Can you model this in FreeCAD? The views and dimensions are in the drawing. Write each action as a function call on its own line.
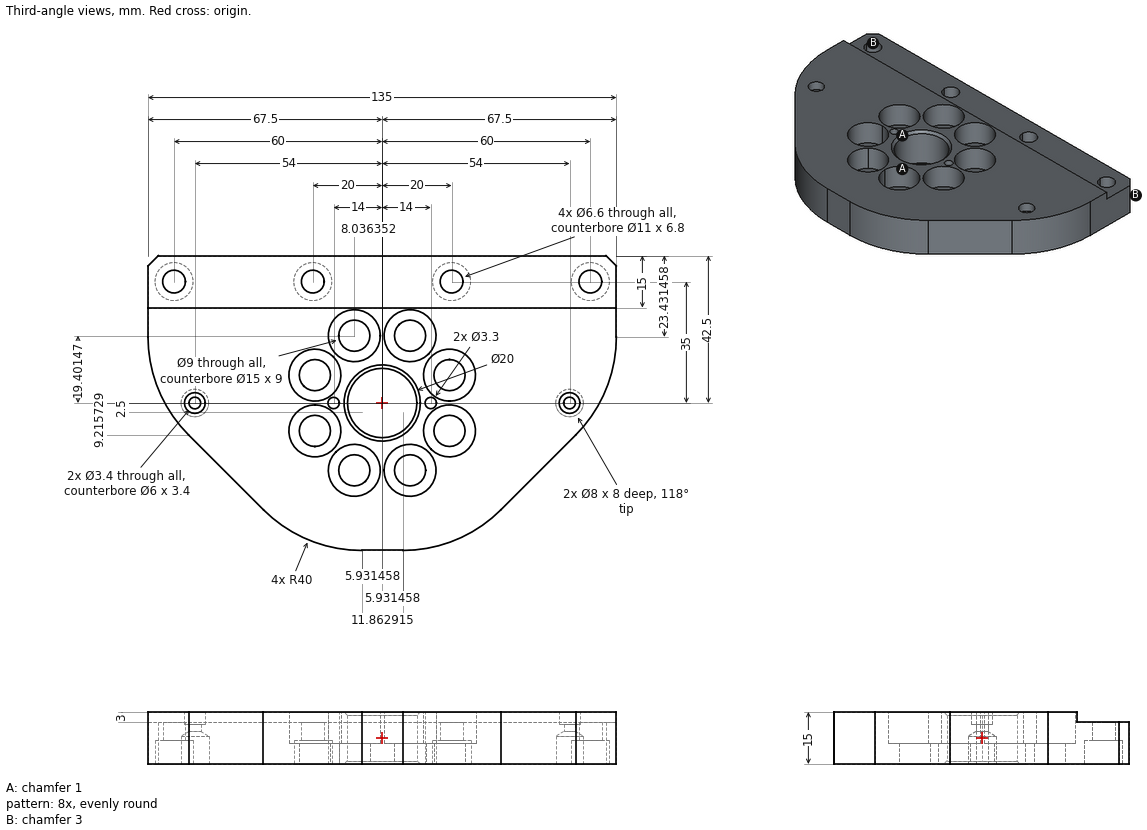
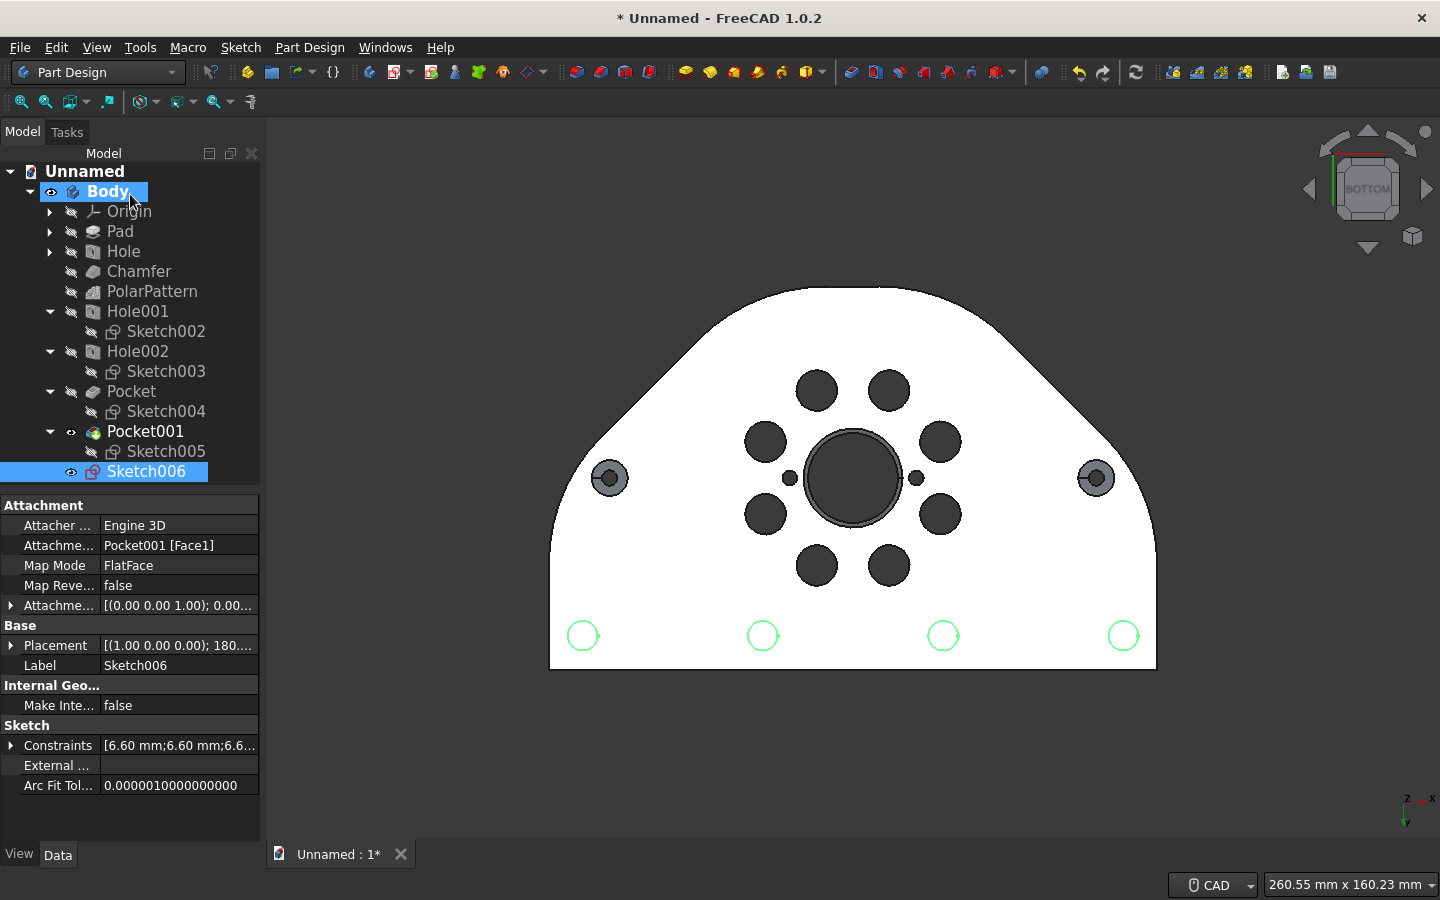
click(876, 72)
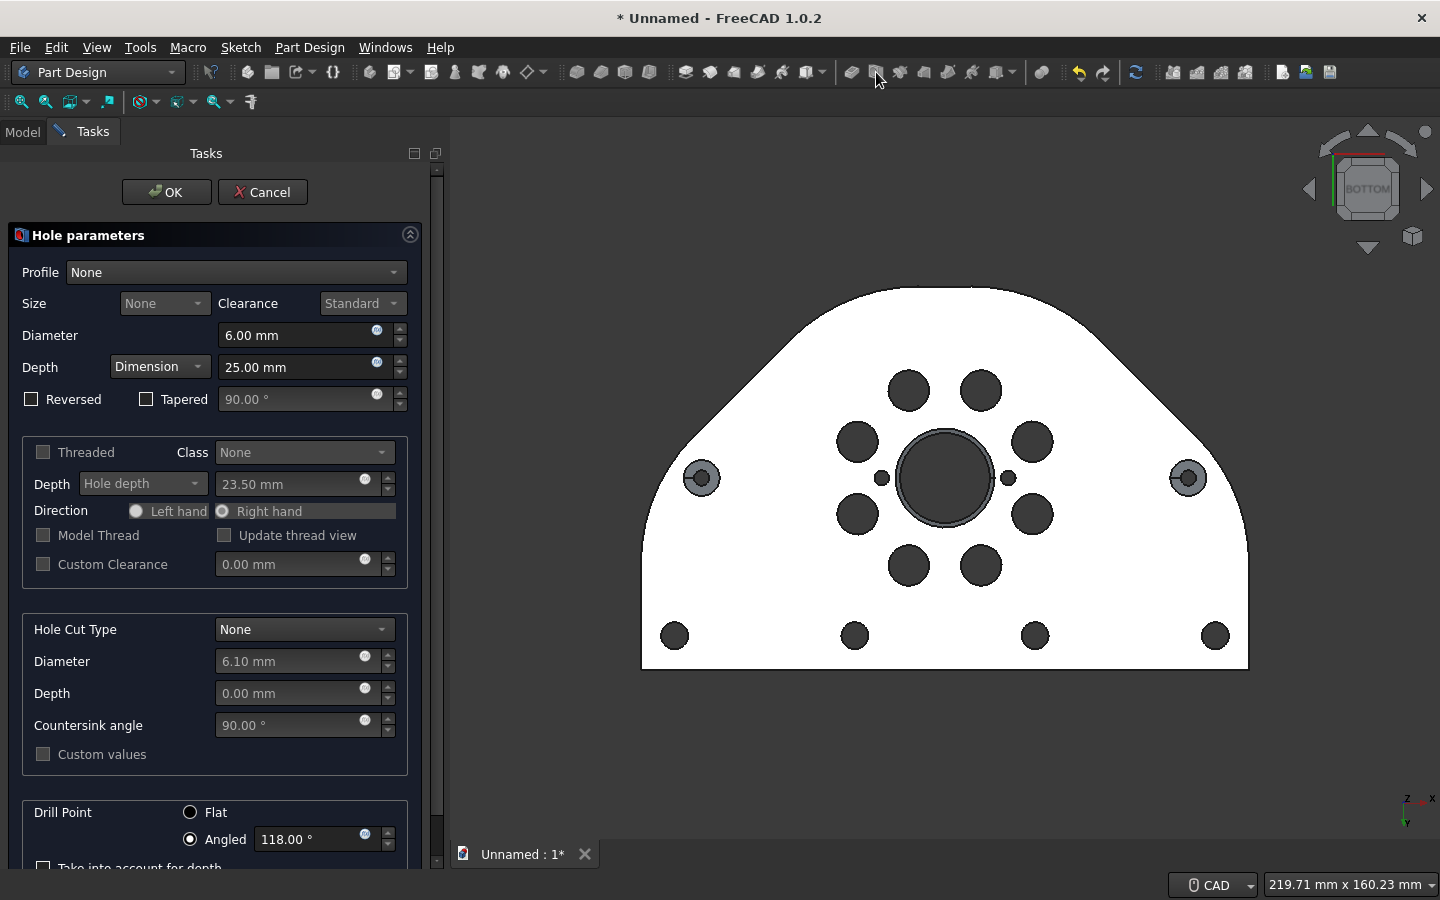
triple_click(305, 335)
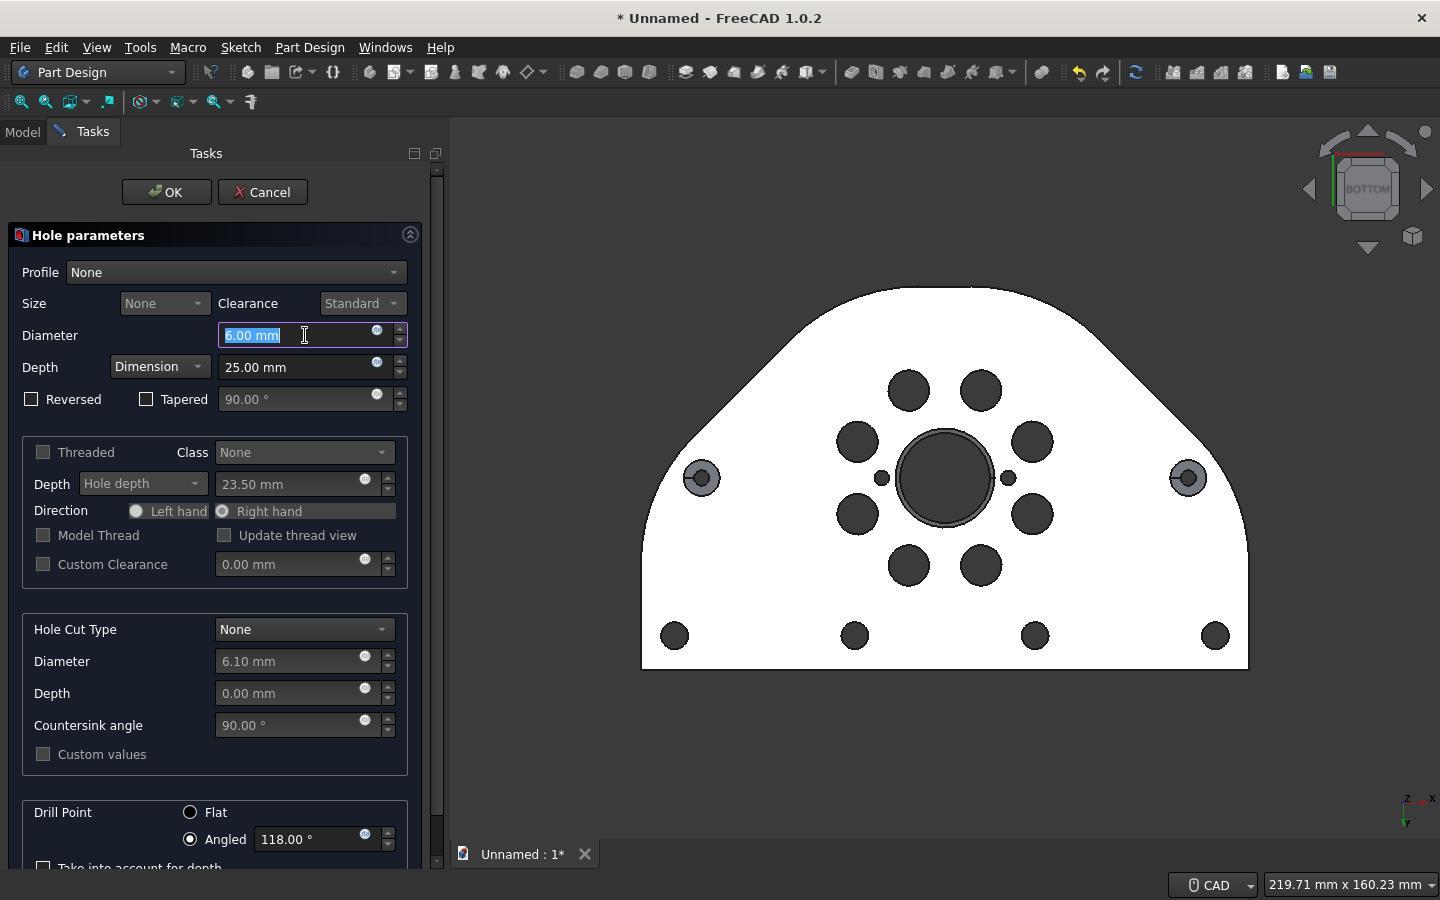
text(6.6)
key(Tab)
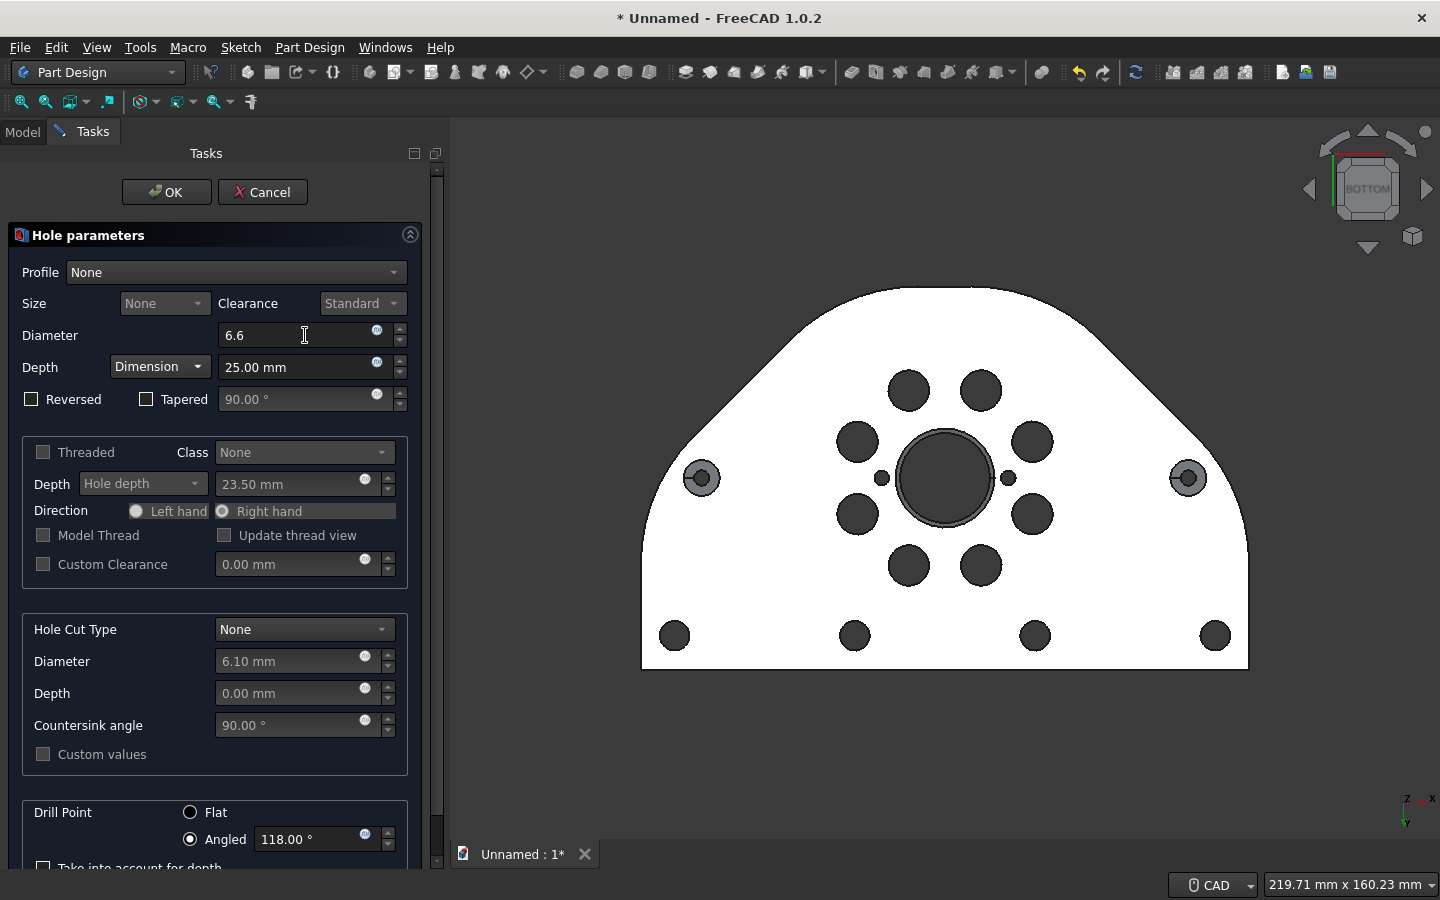
click(161, 366)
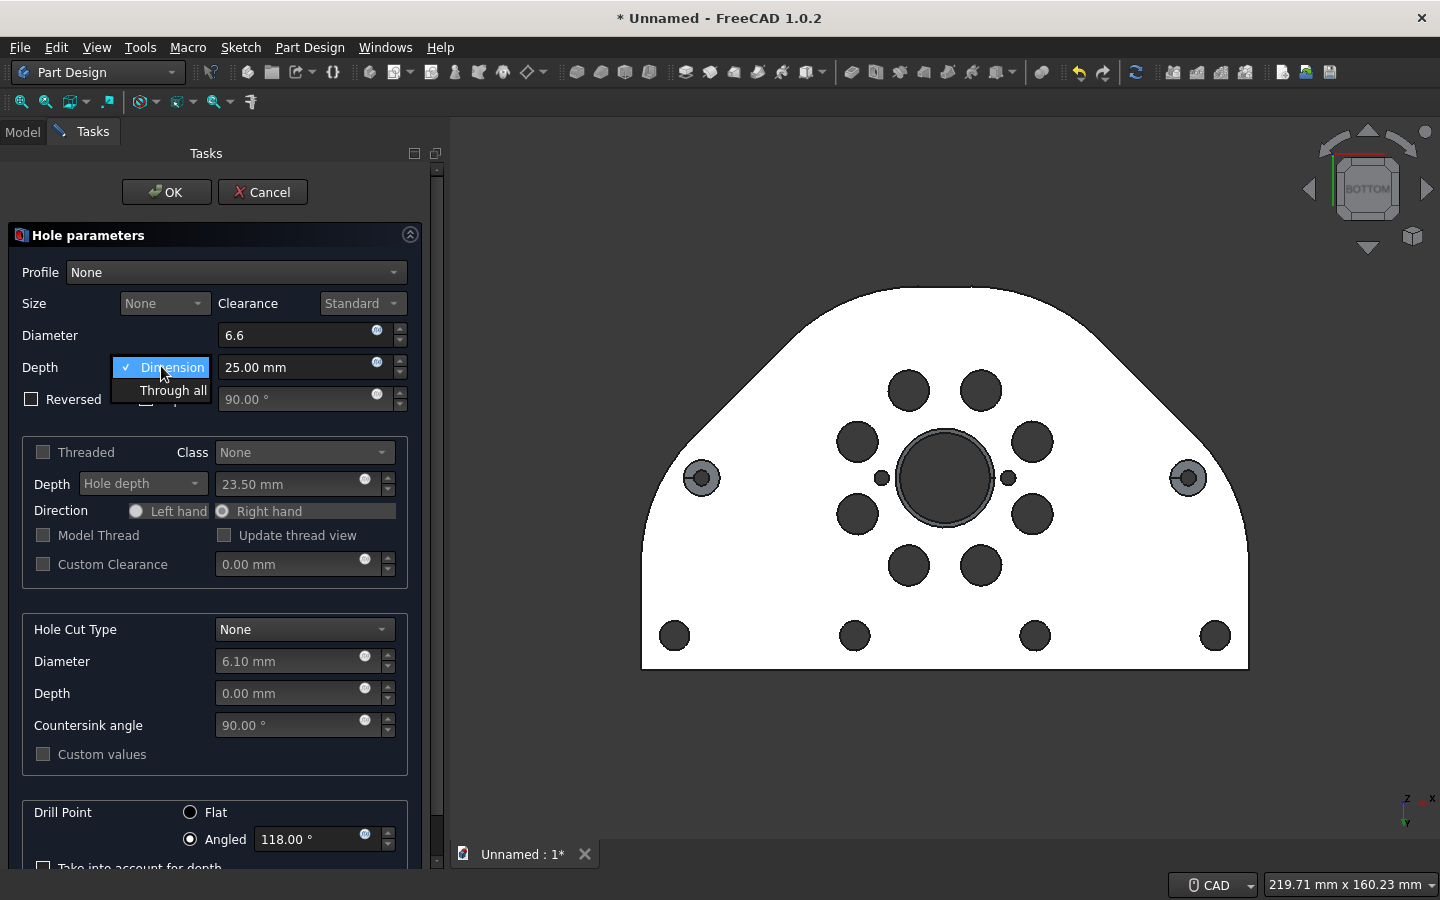
click(160, 390)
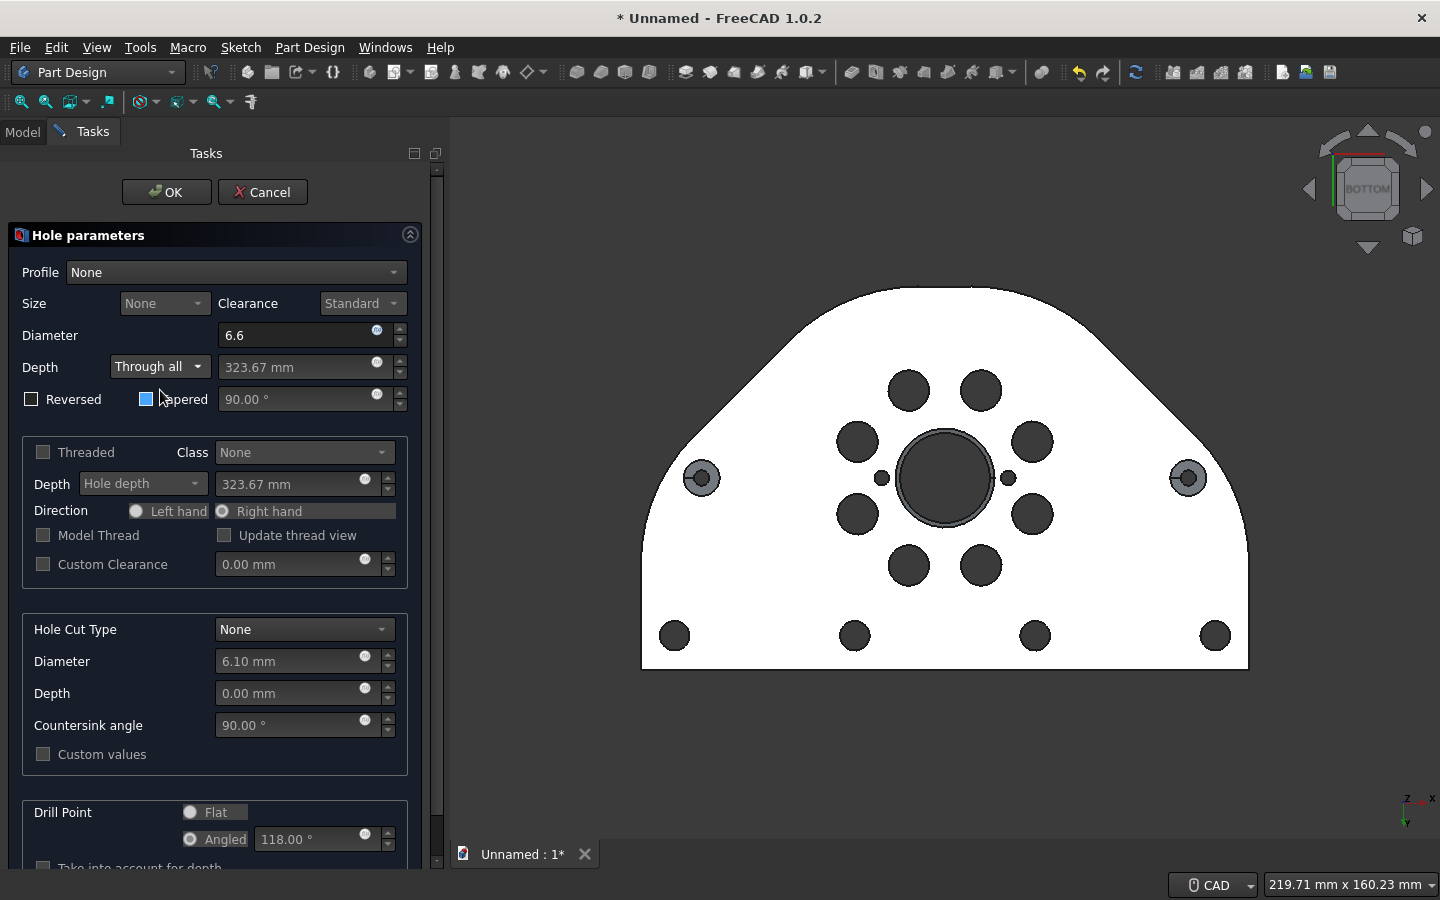
click(306, 630)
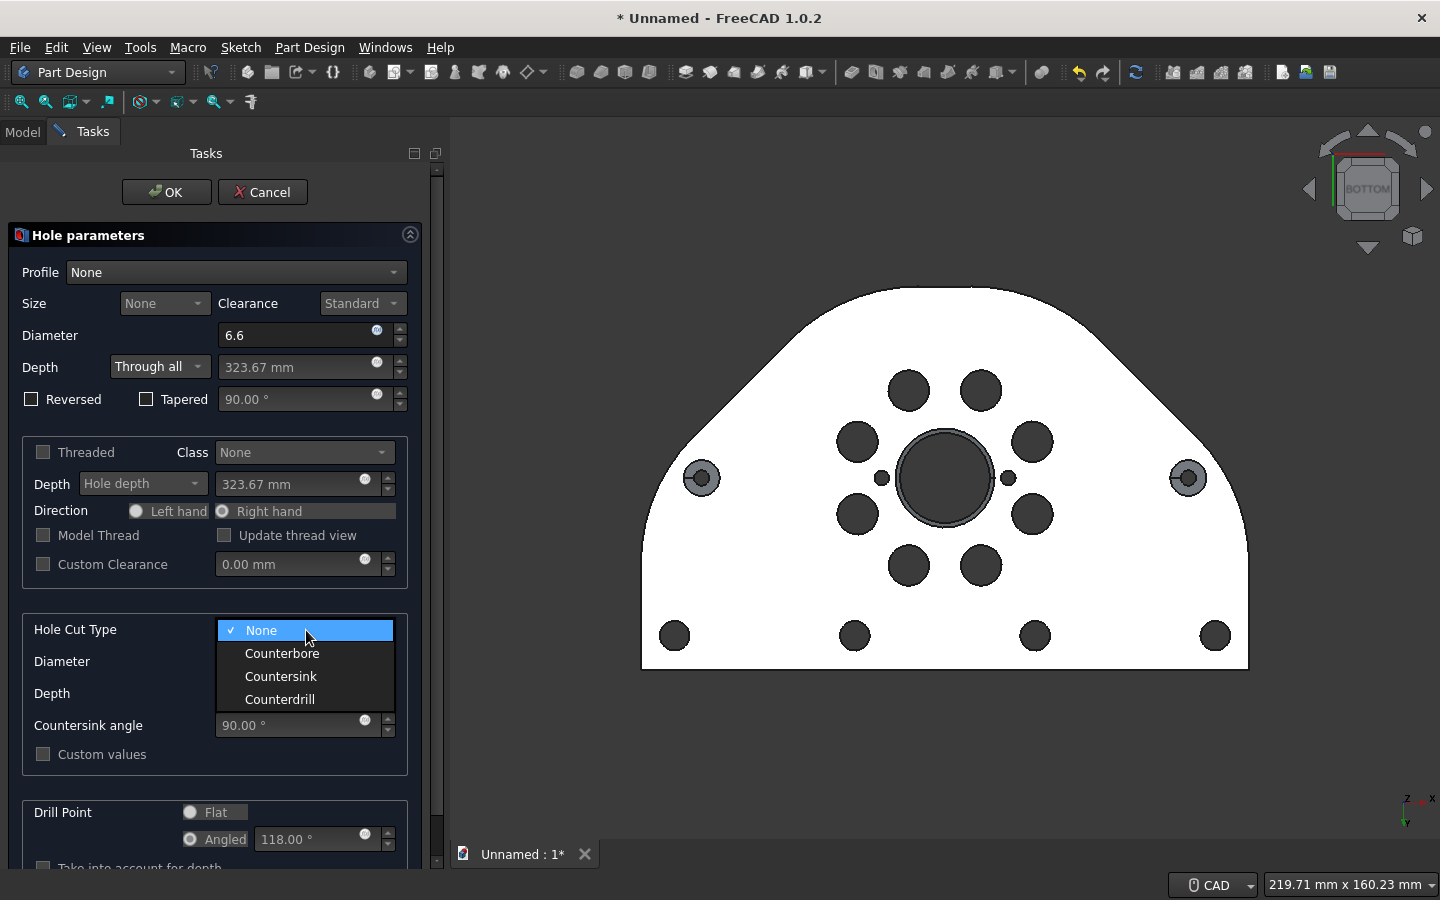
click(304, 654)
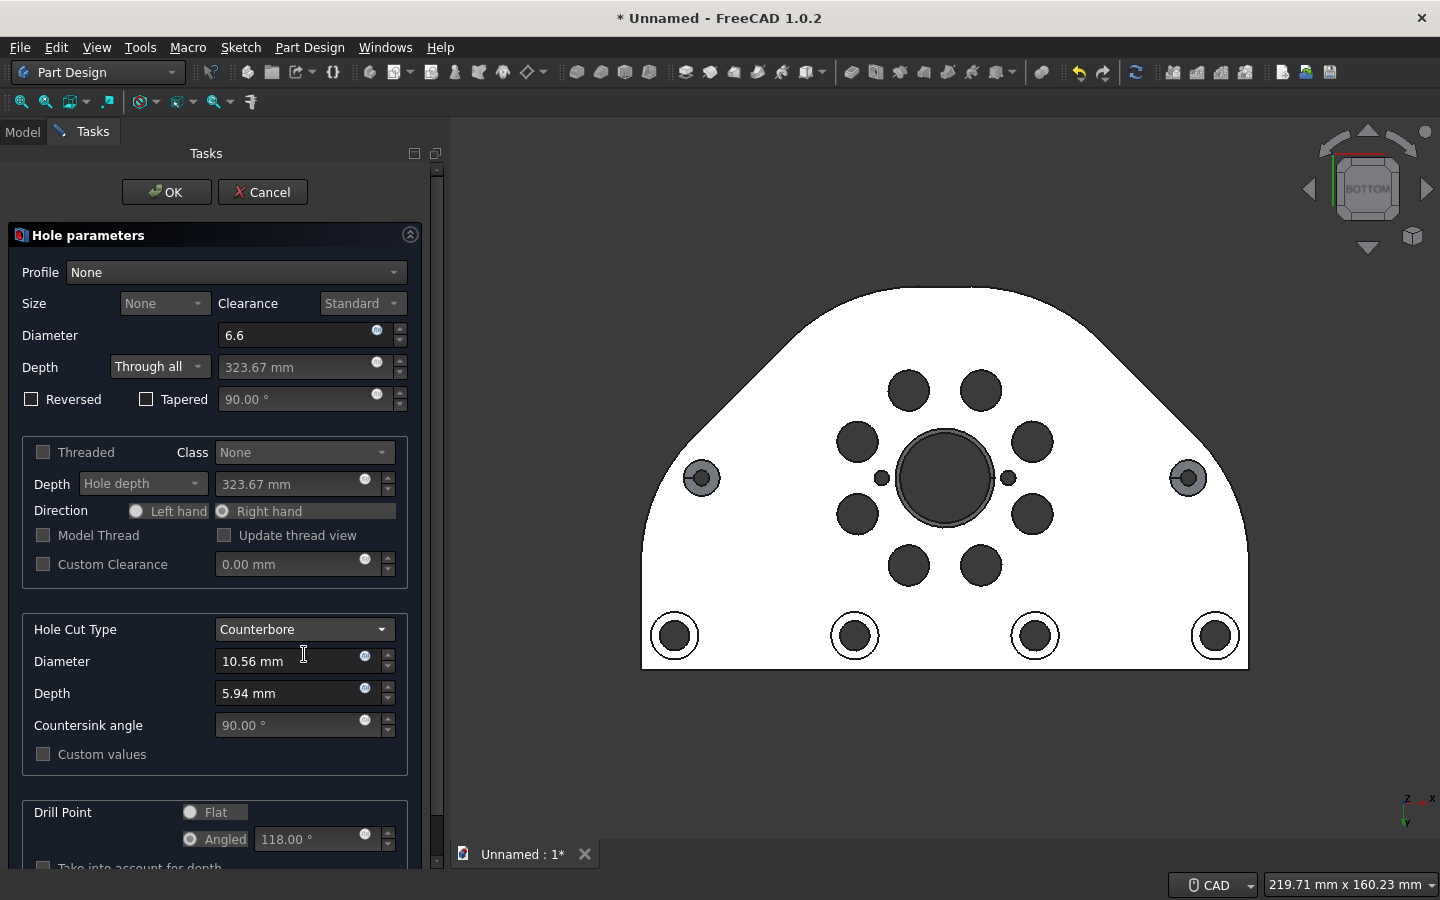
triple_click(298, 661)